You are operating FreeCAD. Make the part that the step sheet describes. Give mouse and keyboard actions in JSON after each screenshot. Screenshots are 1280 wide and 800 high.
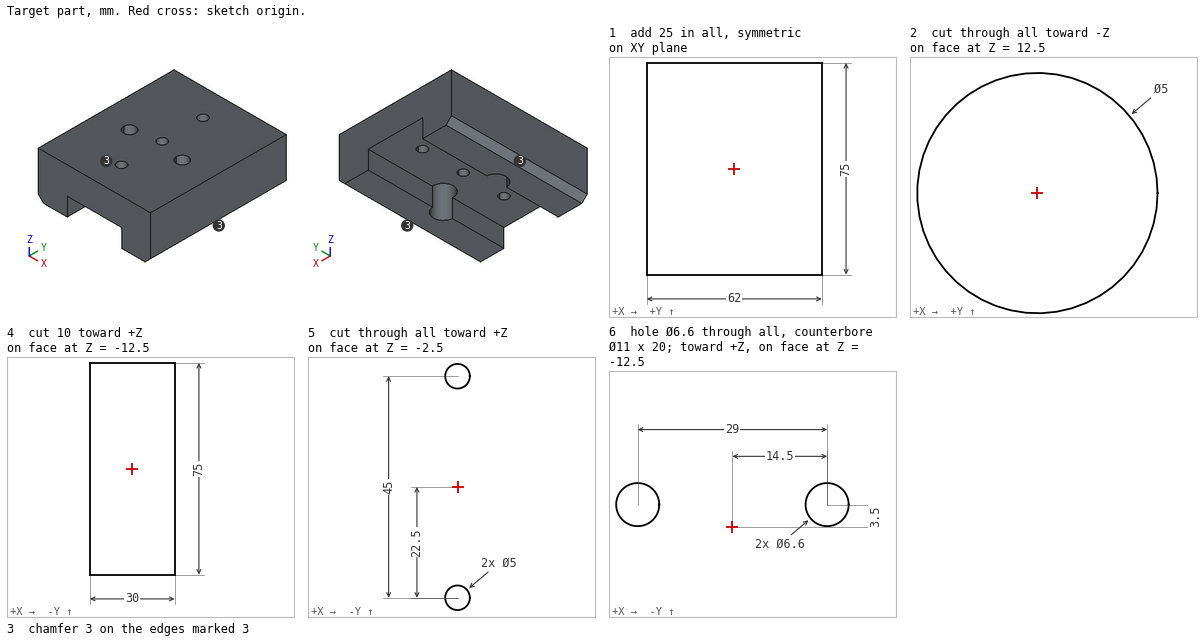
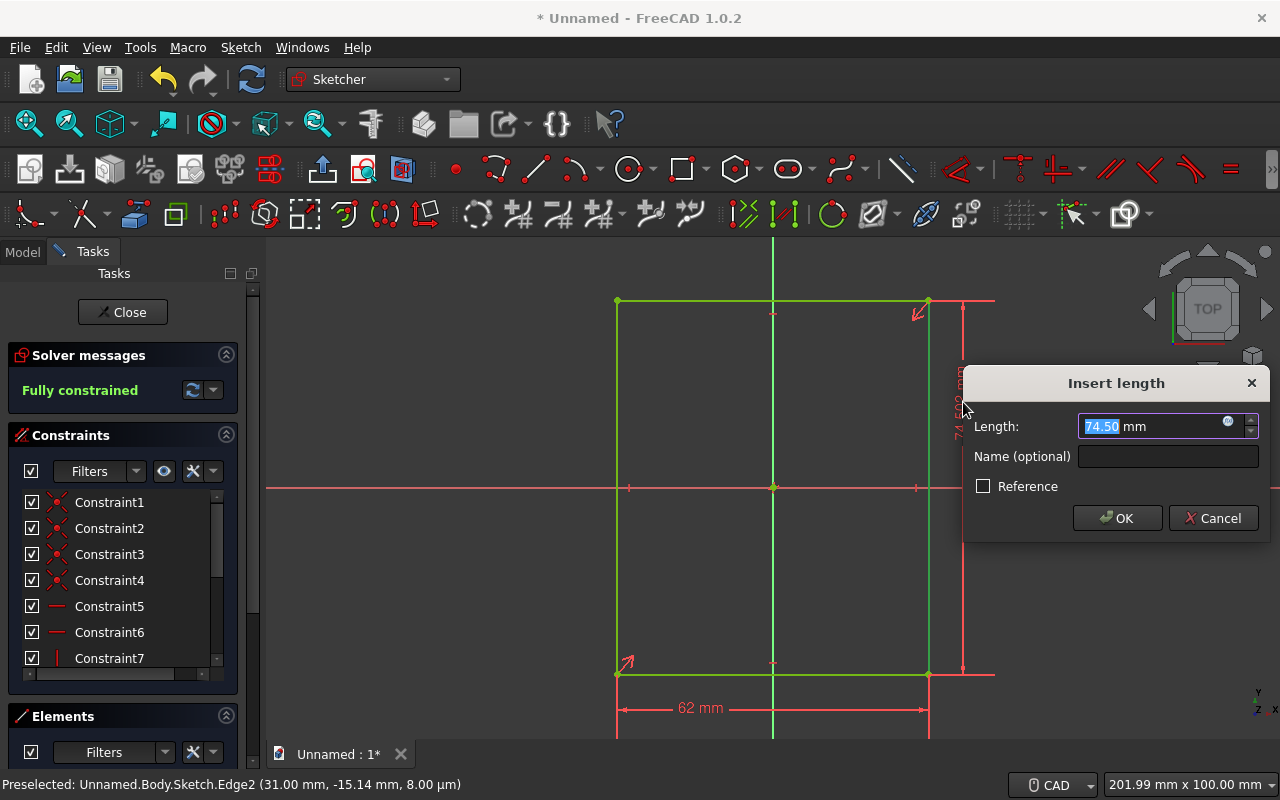
{"action": "type", "text": "75"}
{"action": "key", "text": "Return"}
{"action": "key", "text": "Escape"}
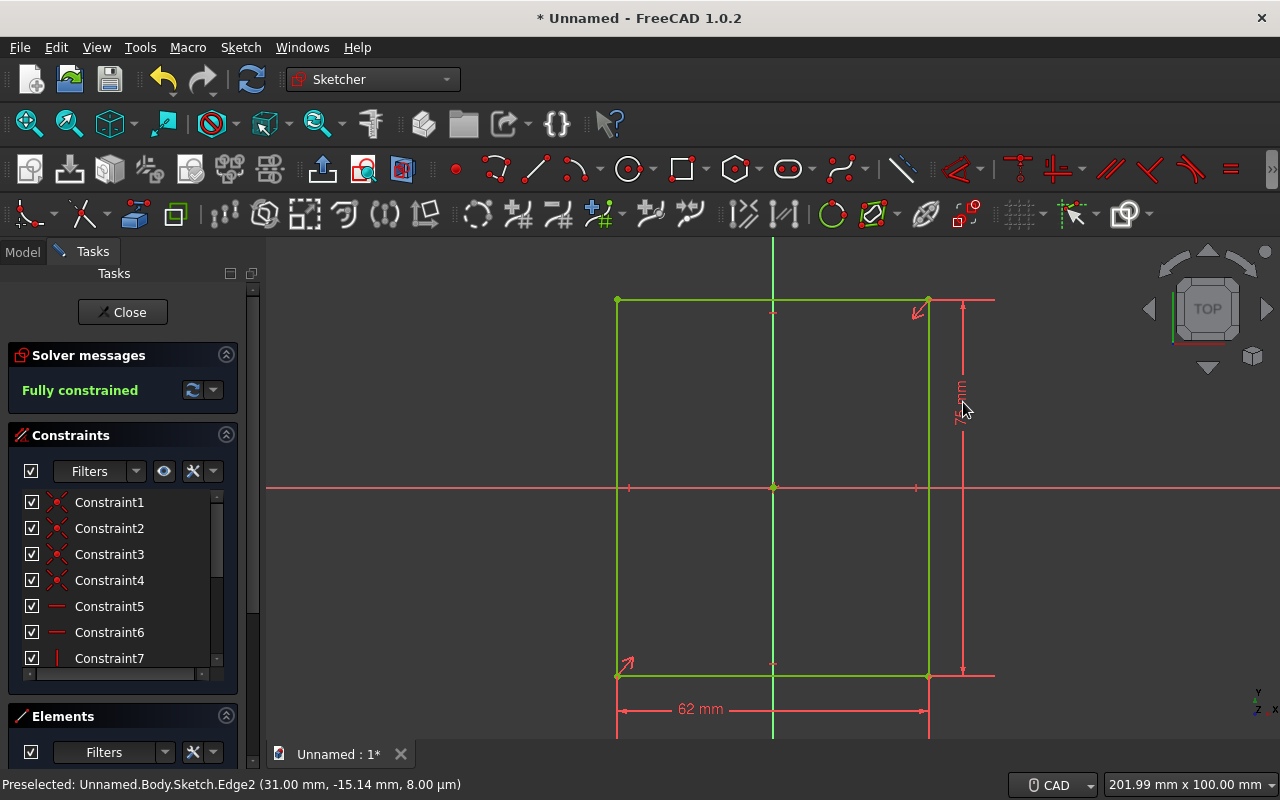
{"action": "left_click", "coordinate": [123, 312]}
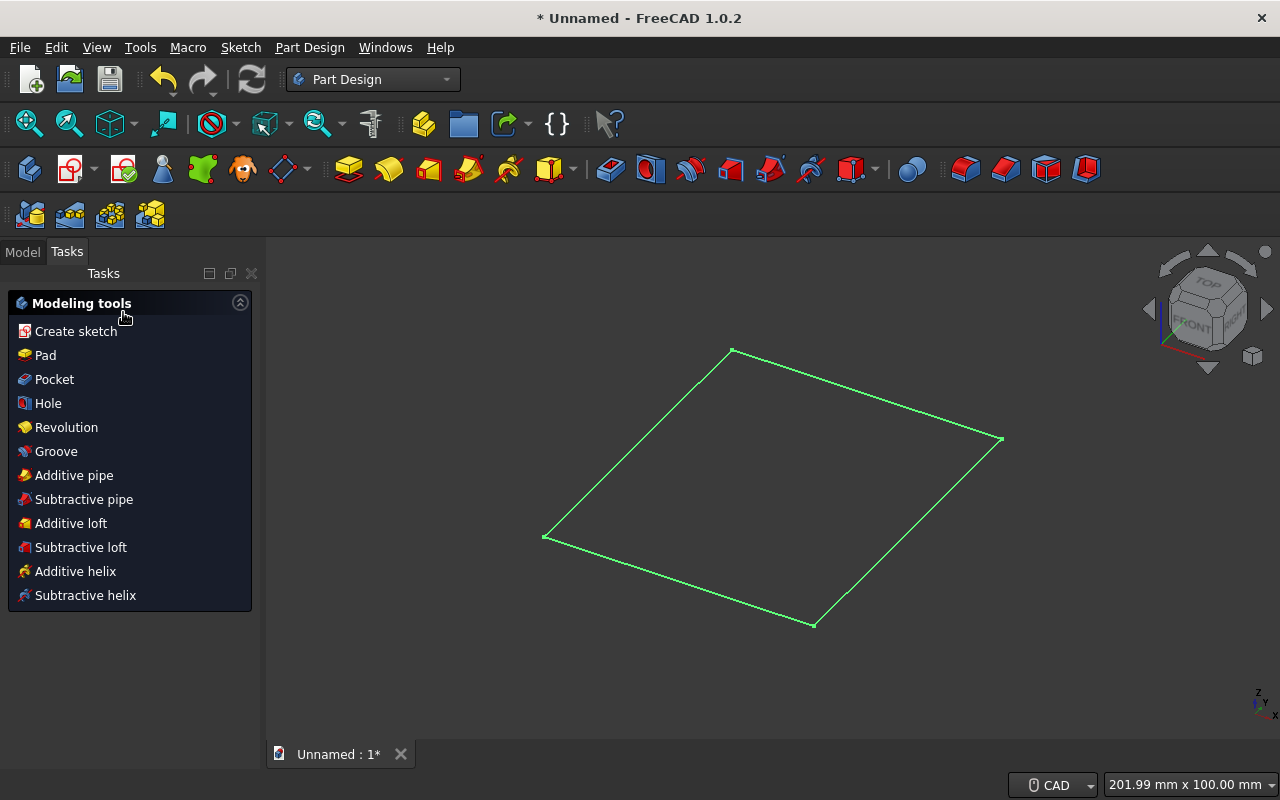
{"action": "left_click", "coordinate": [350, 170]}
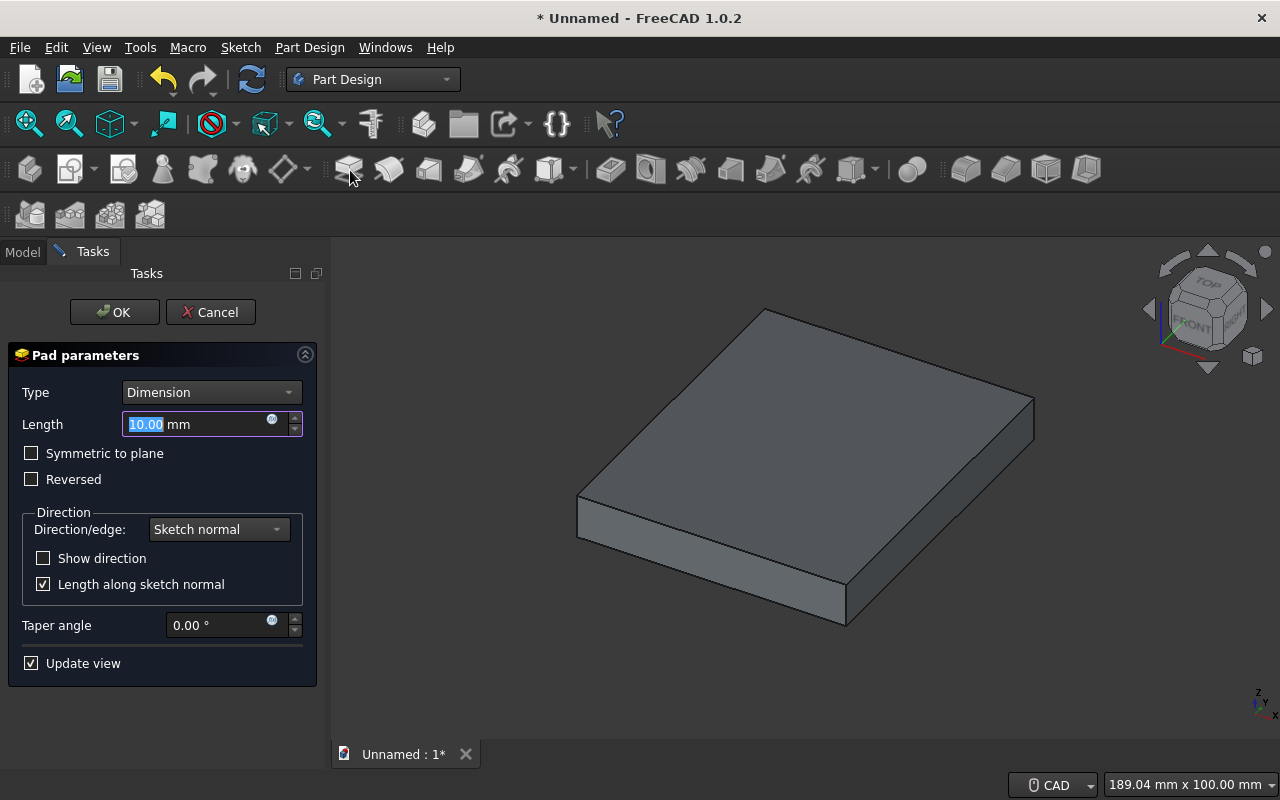
{"action": "type", "text": "25"}
{"action": "key", "text": "Tab"}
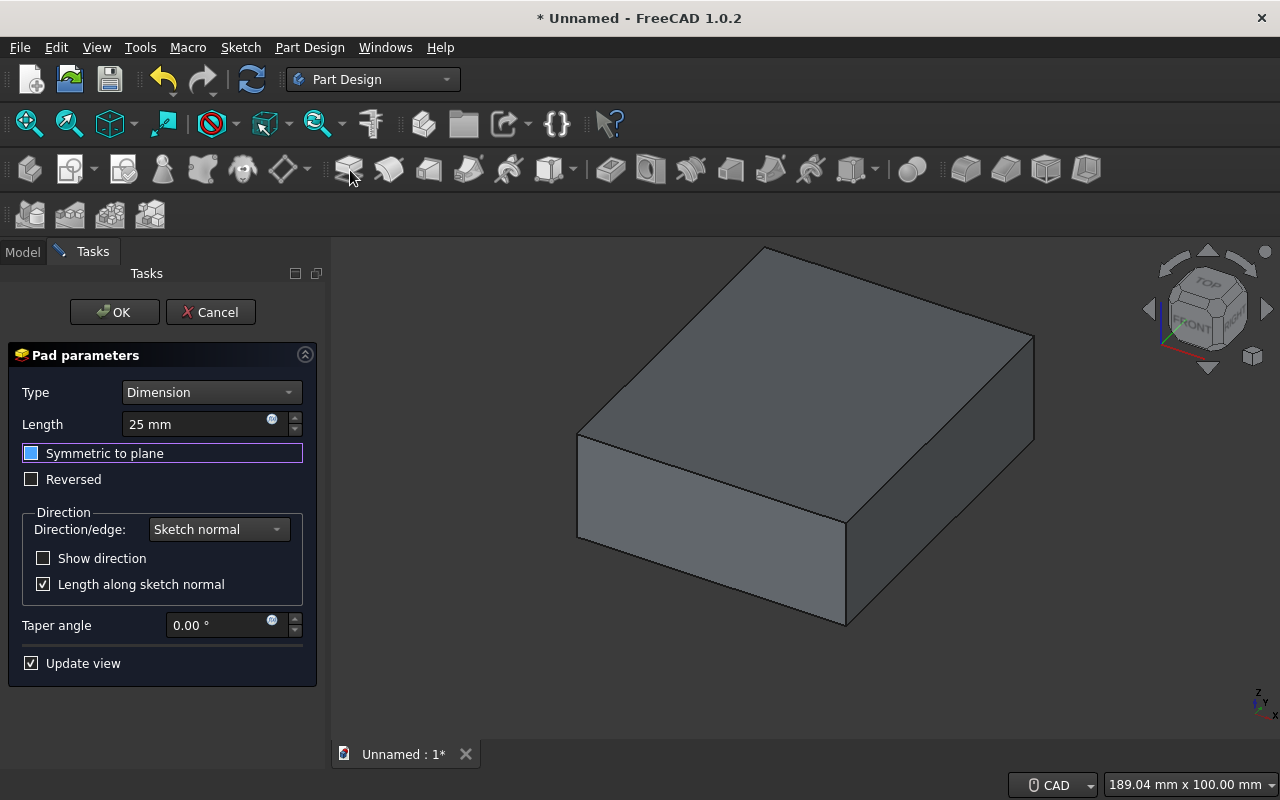
{"action": "left_click", "coordinate": [30, 453]}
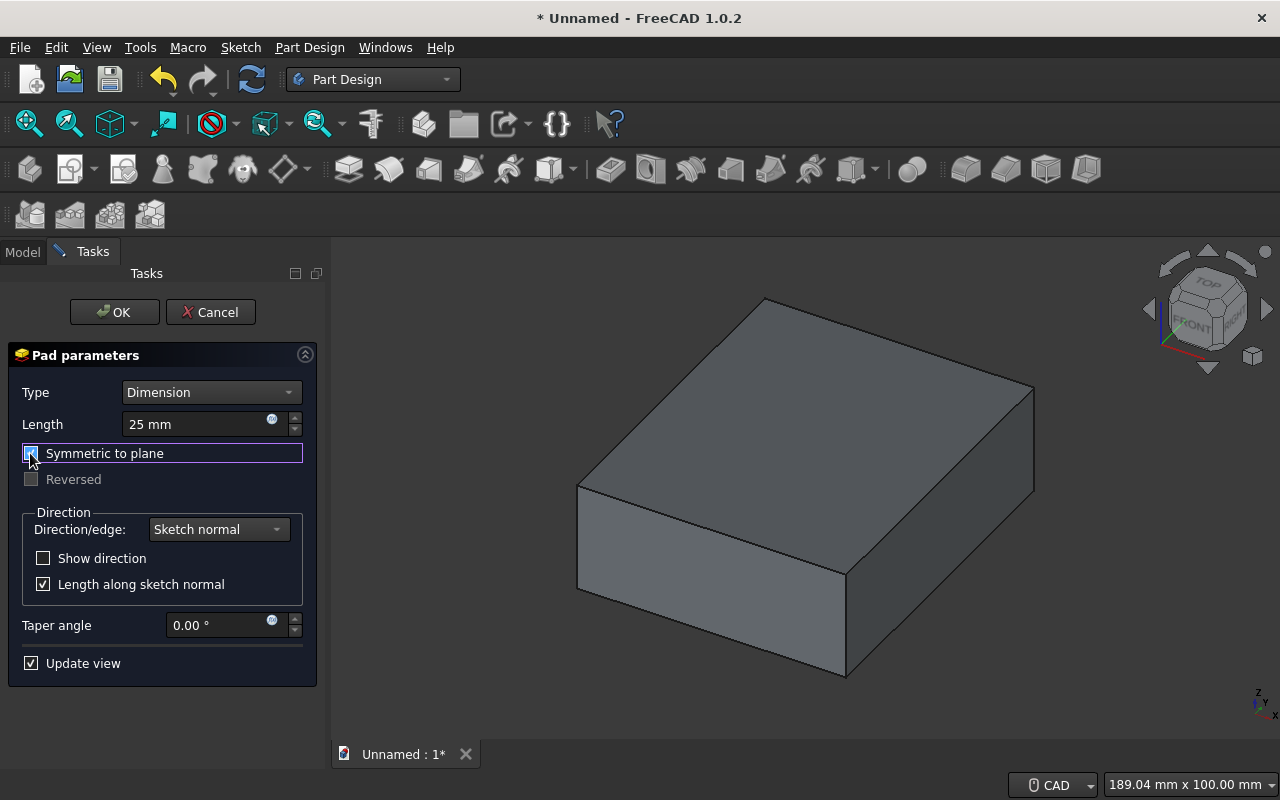
{"action": "left_click", "coordinate": [115, 312]}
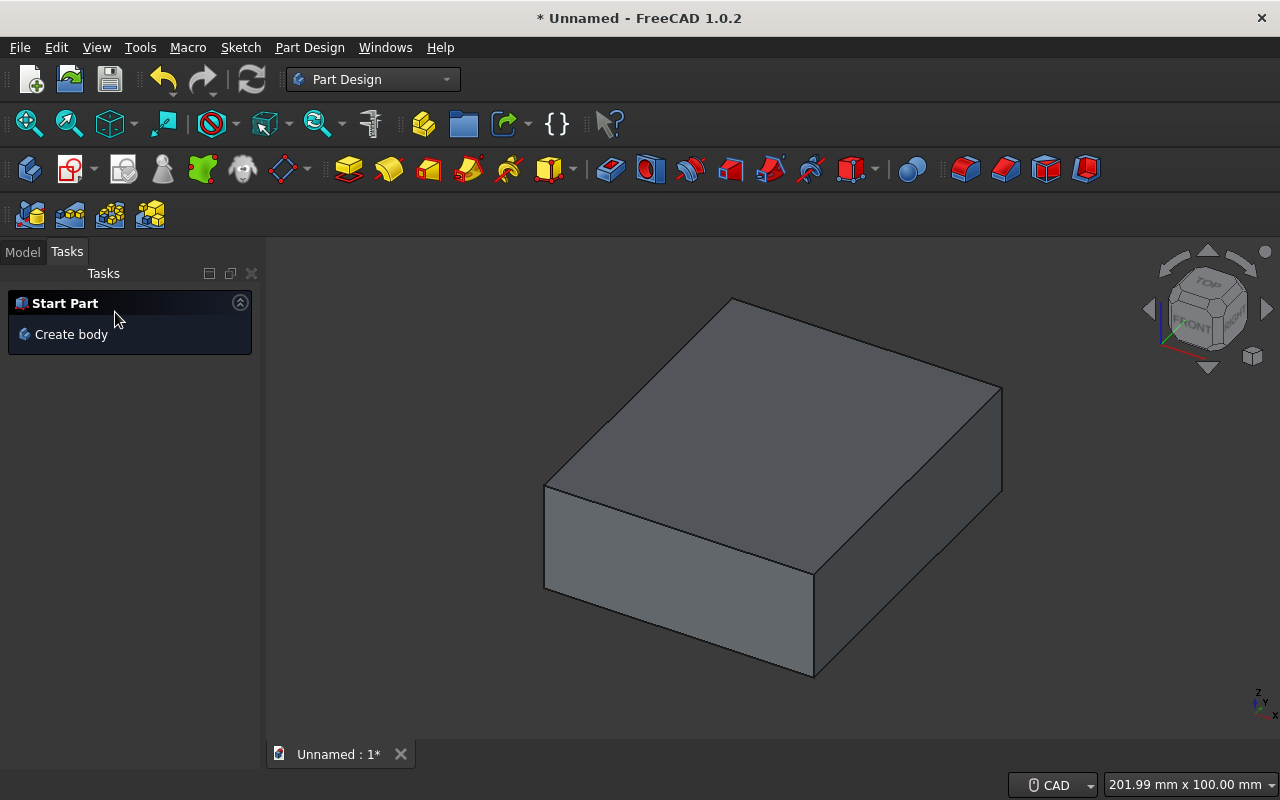
{"action": "left_click", "coordinate": [773, 436]}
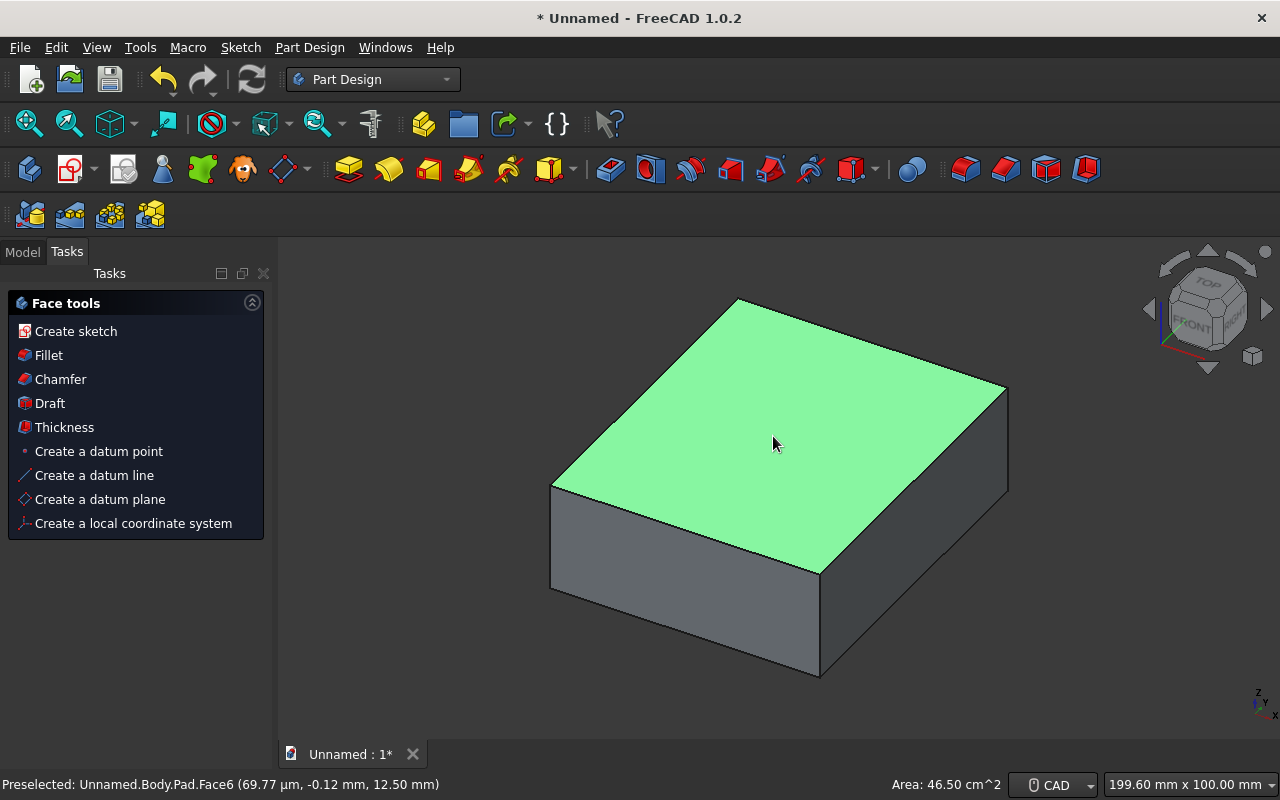
{"action": "left_click", "coordinate": [70, 170]}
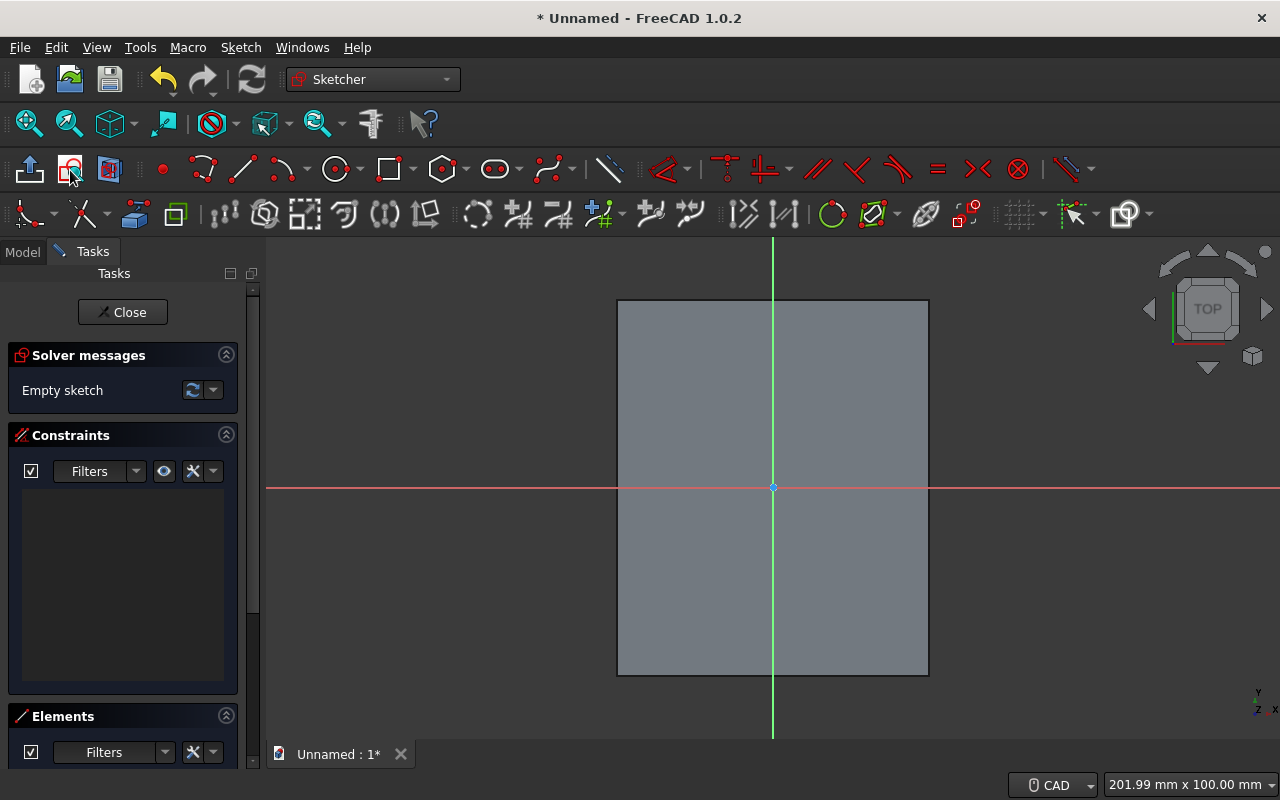
{"action": "scroll", "coordinate": [778, 488], "scroll_direction": "up", "scroll_amount": 13}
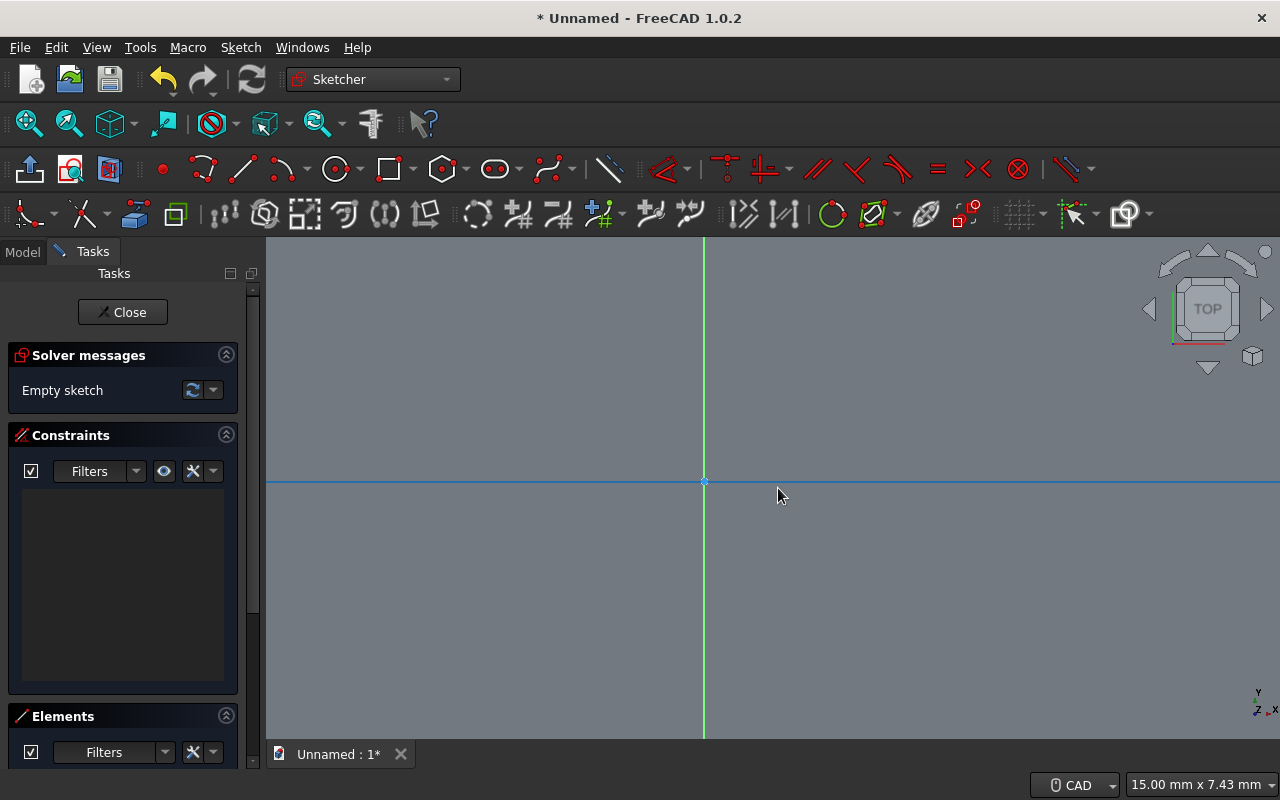
{"action": "key", "text": "g c"}